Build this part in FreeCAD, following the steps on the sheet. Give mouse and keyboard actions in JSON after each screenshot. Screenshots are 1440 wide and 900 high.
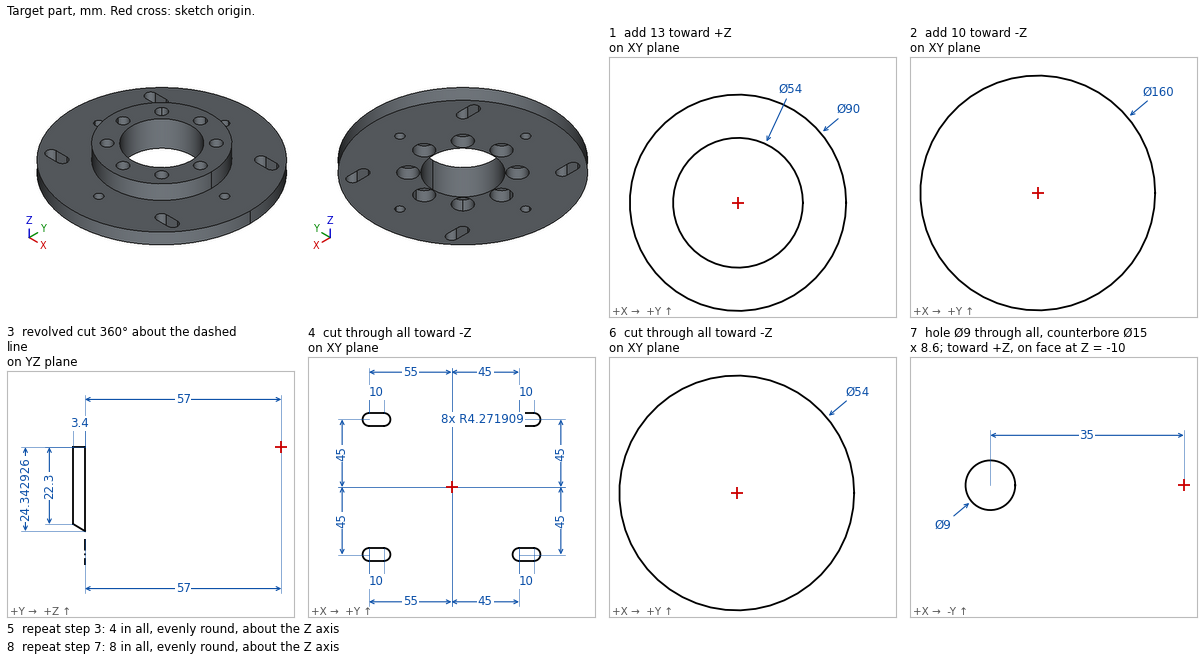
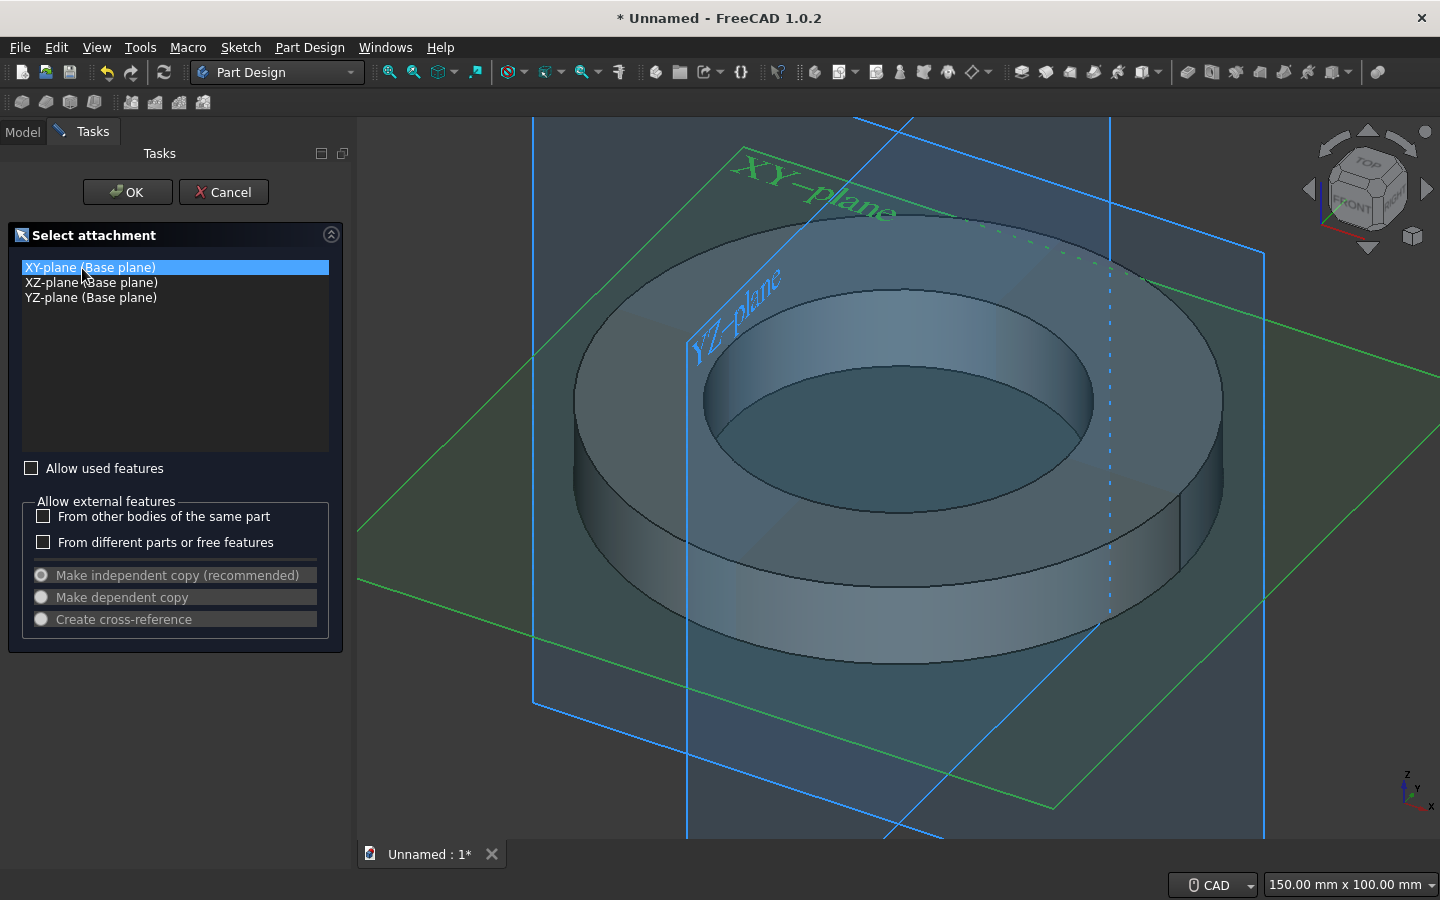
{"action": "left_click", "coordinate": [128, 192]}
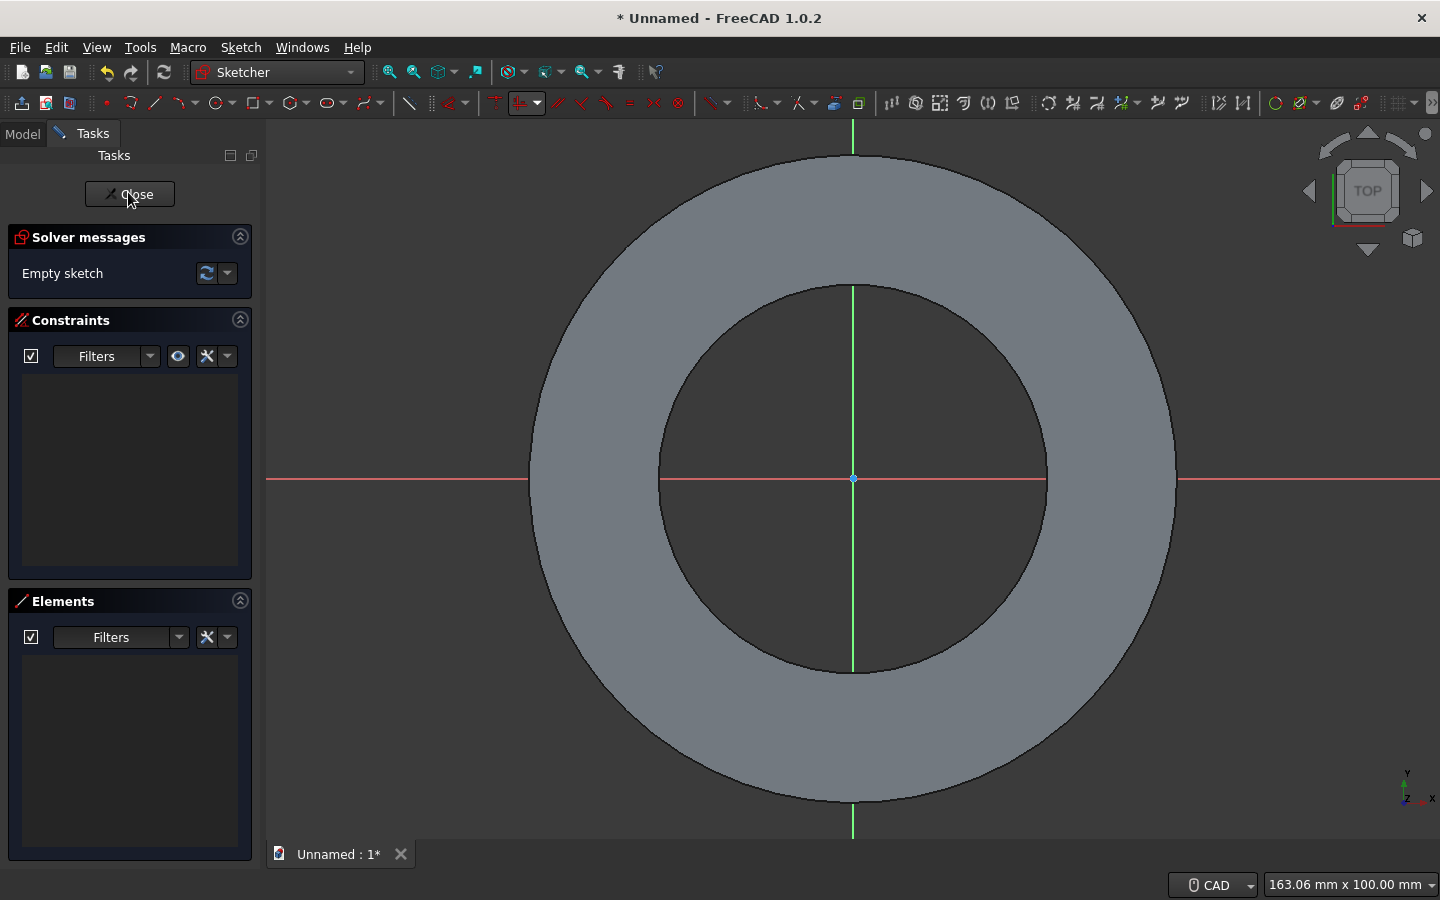
{"action": "key", "text": "q s"}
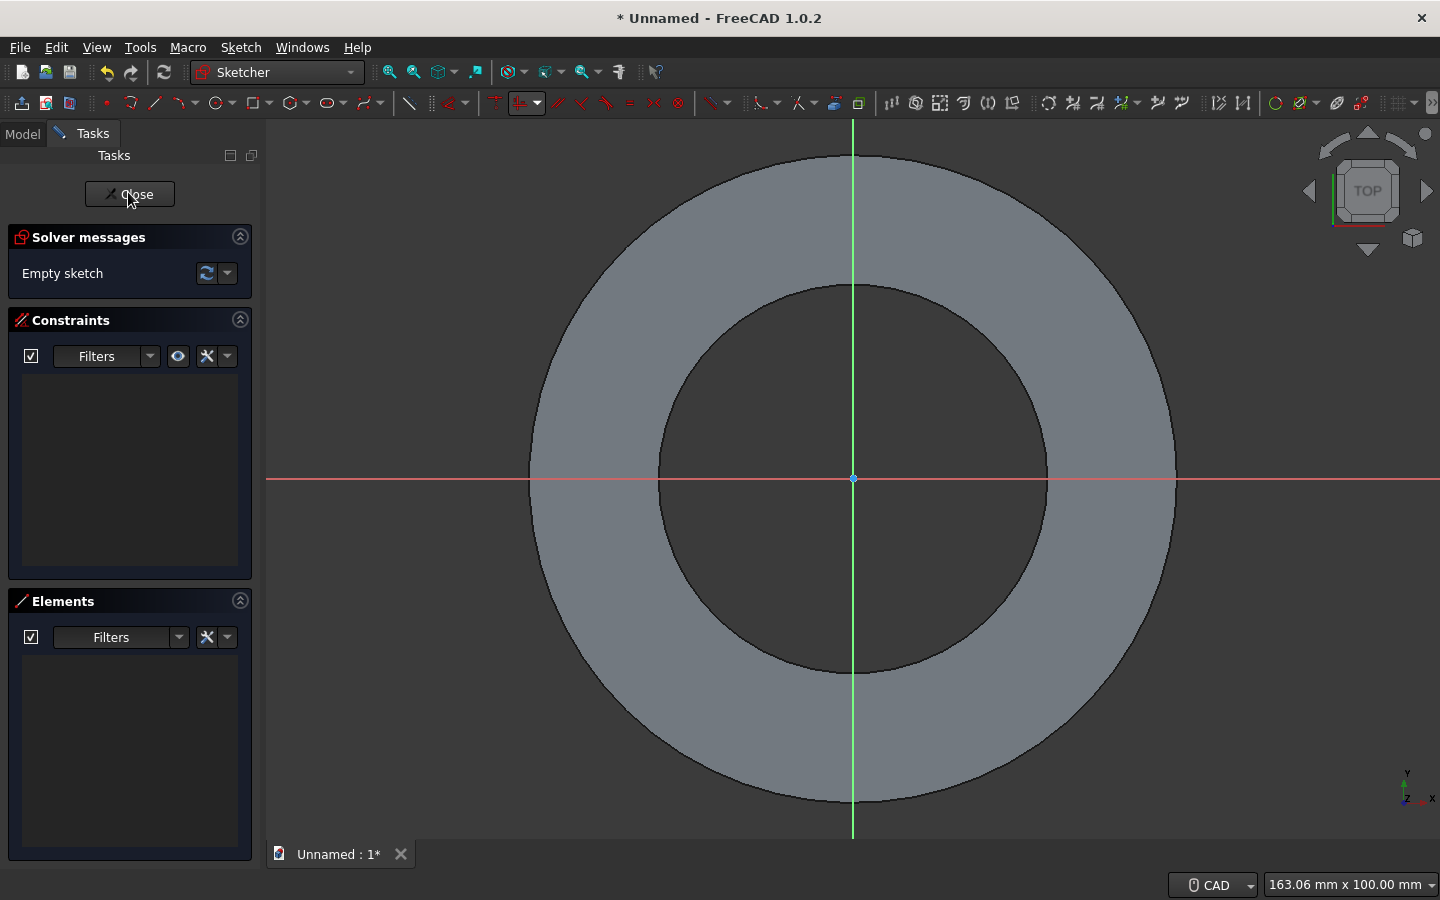
{"action": "scroll", "coordinate": [729, 479], "scroll_direction": "down", "scroll_amount": 4}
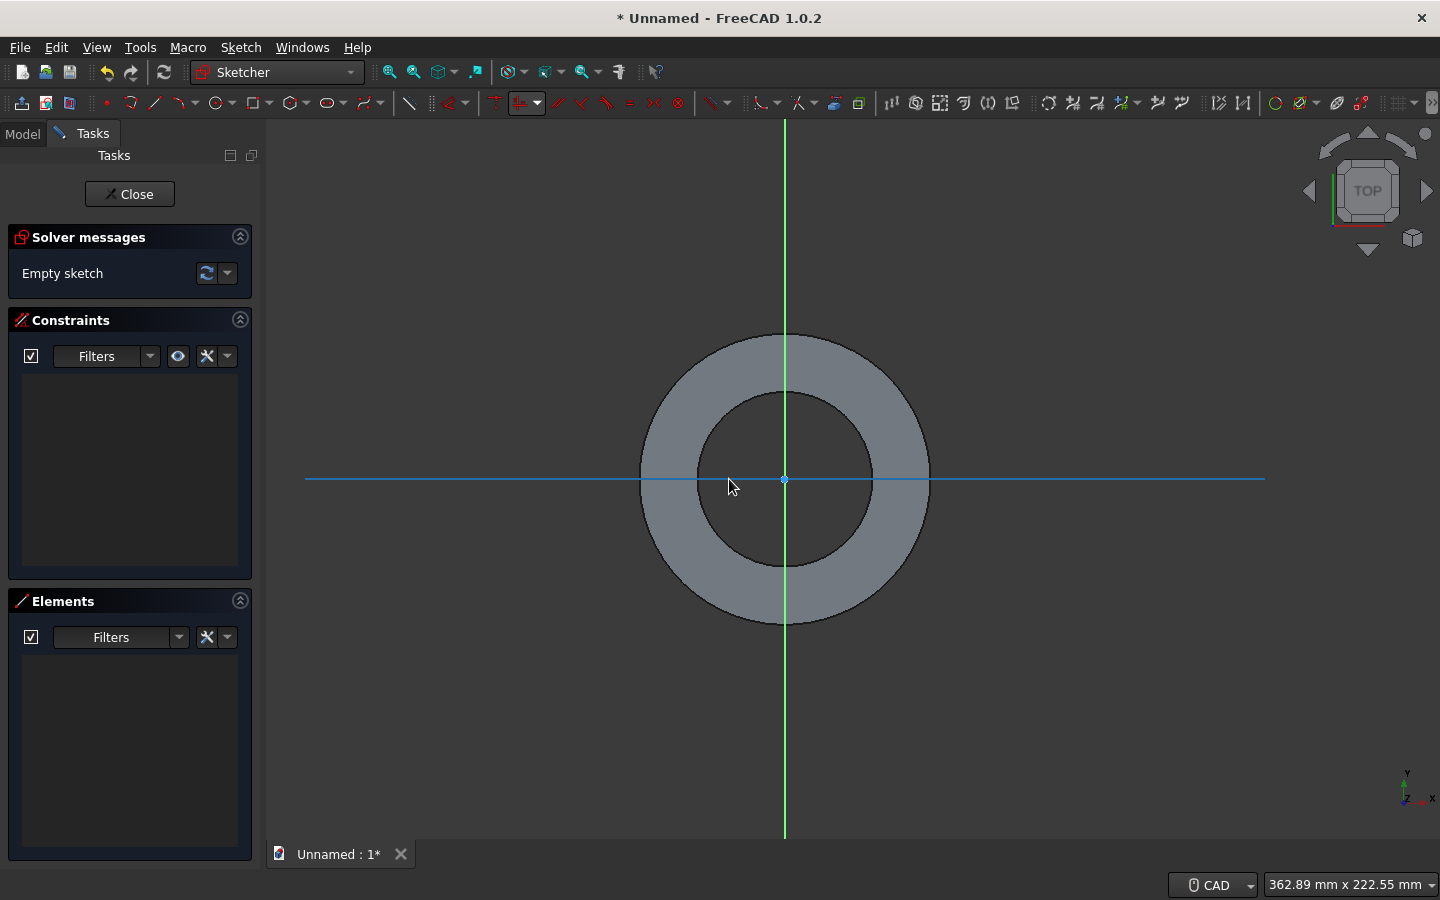
{"action": "left_click", "coordinate": [216, 104]}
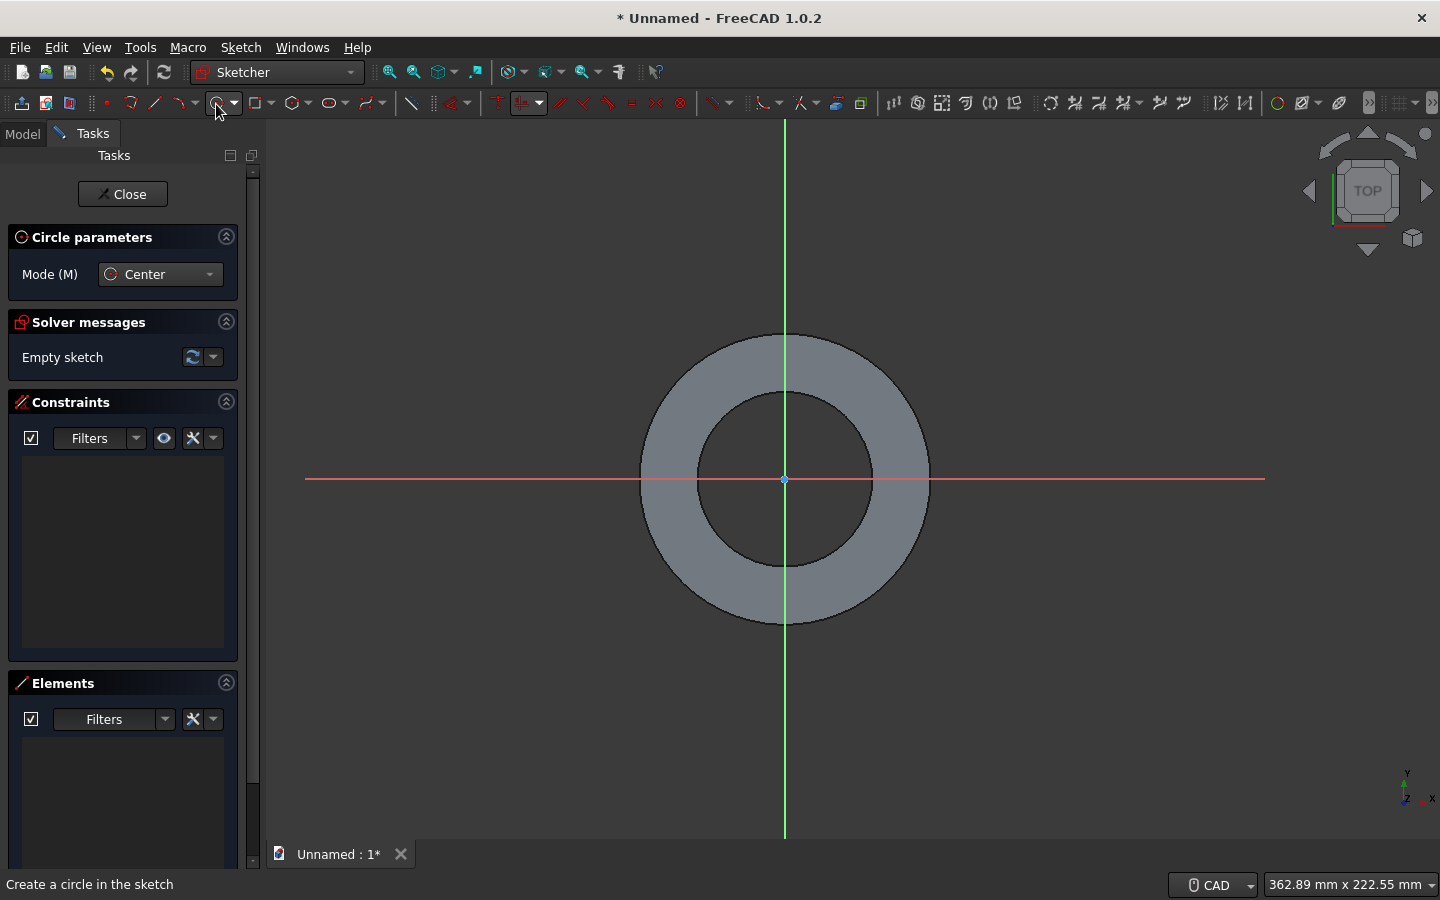
{"action": "left_click", "coordinate": [785, 479]}
{"action": "mouse_move", "coordinate": [968, 296]}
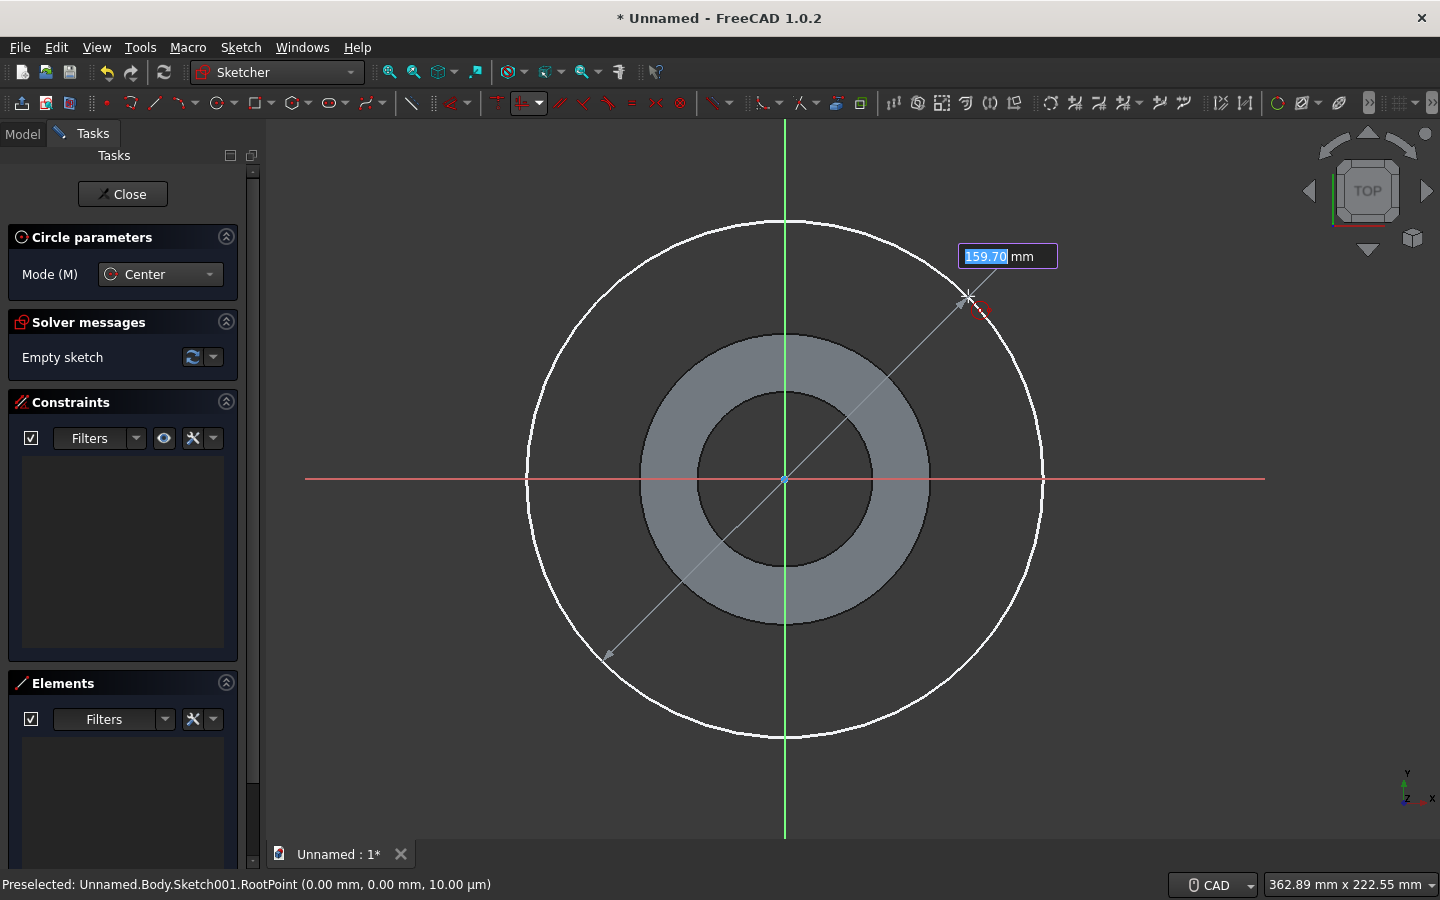
{"action": "type", "text": "160"}
{"action": "key", "text": "Return"}
{"action": "key", "text": "Escape"}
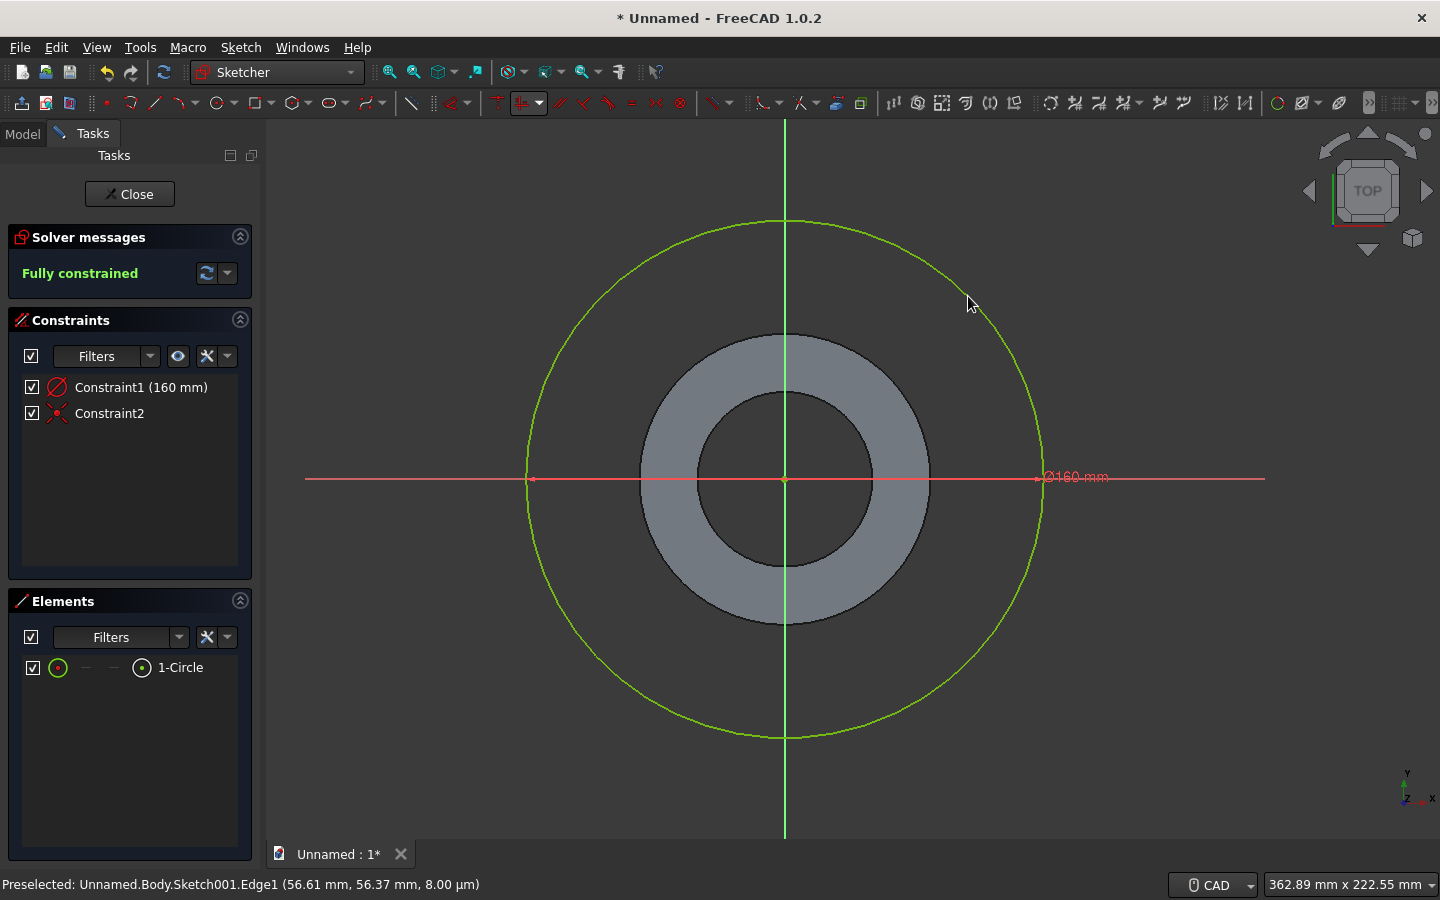
{"action": "left_click", "coordinate": [130, 194]}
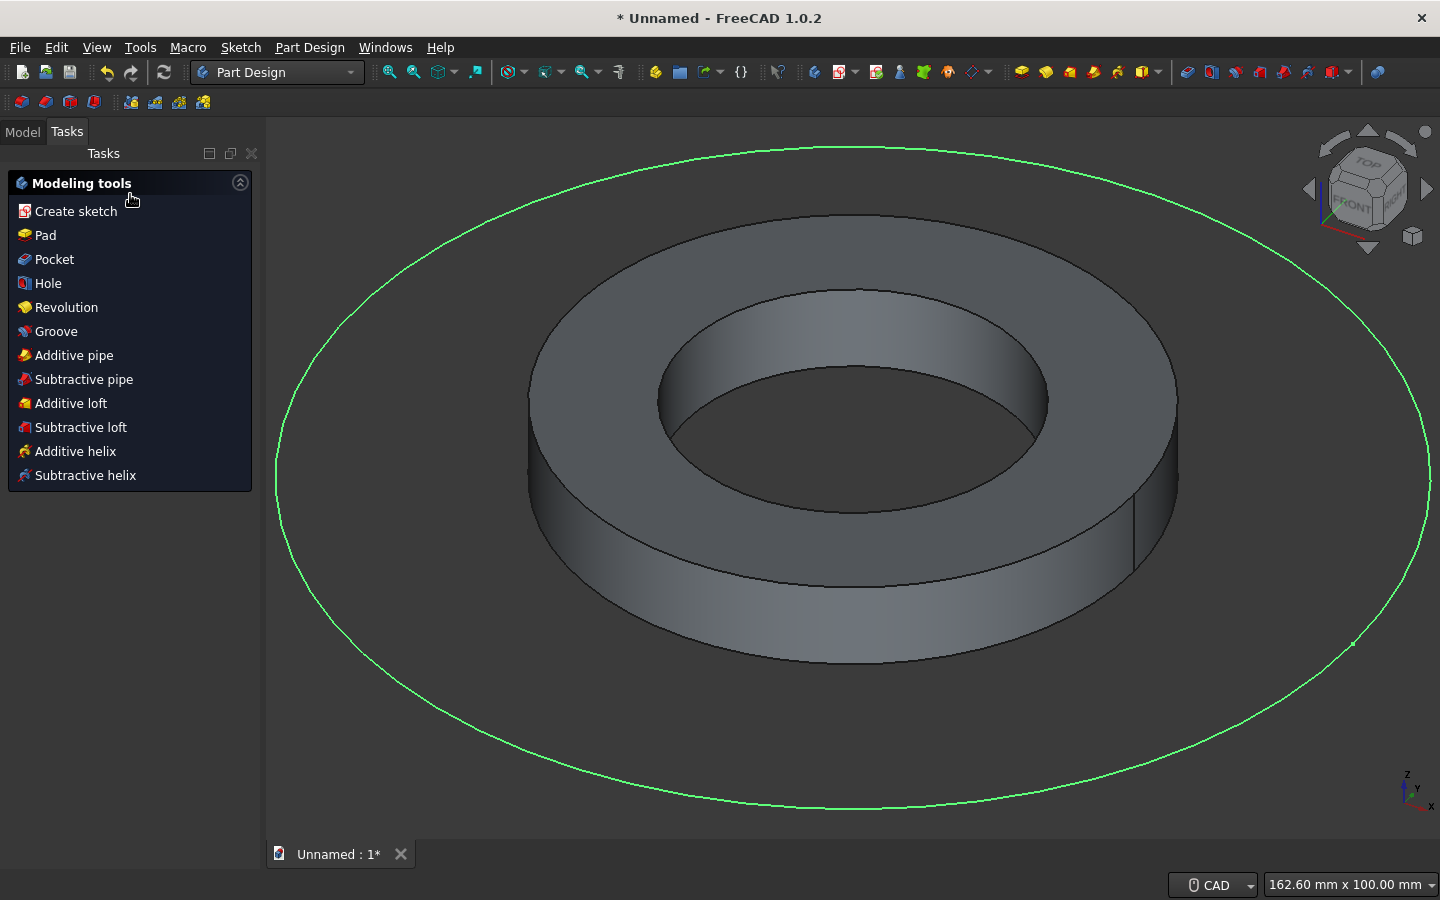
{"action": "left_click", "coordinate": [1022, 72]}